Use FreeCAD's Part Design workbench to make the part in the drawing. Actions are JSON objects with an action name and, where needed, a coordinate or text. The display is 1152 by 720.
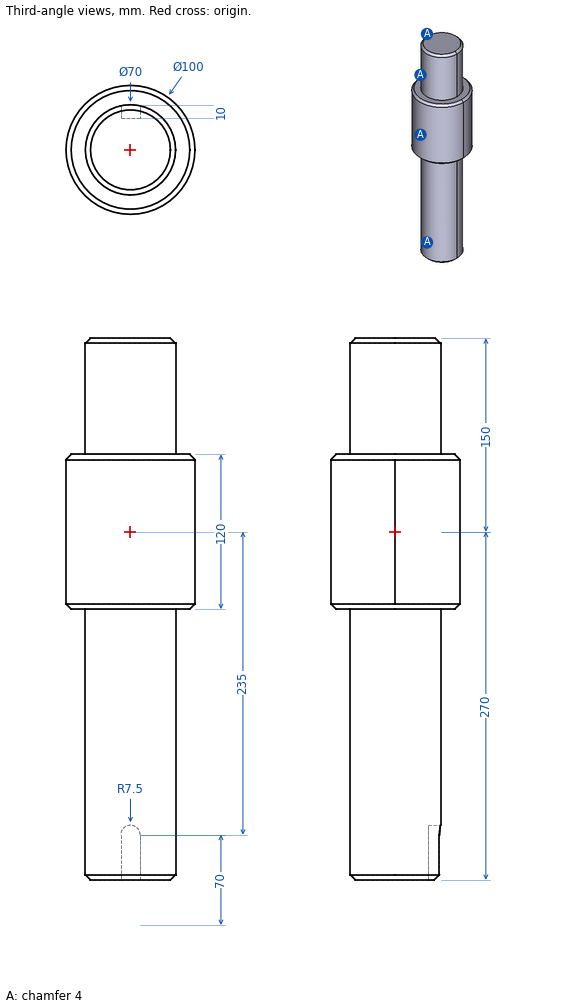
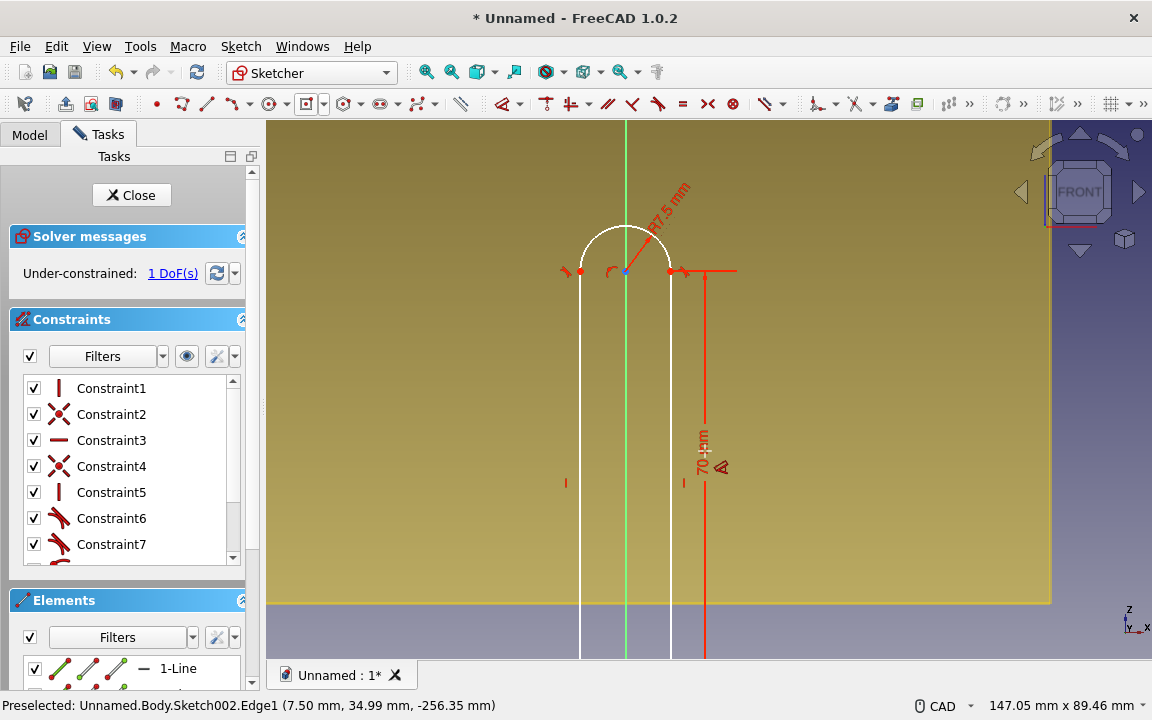
{"action": "left_click", "coordinate": [671, 271]}
{"action": "left_click", "coordinate": [705, 181]}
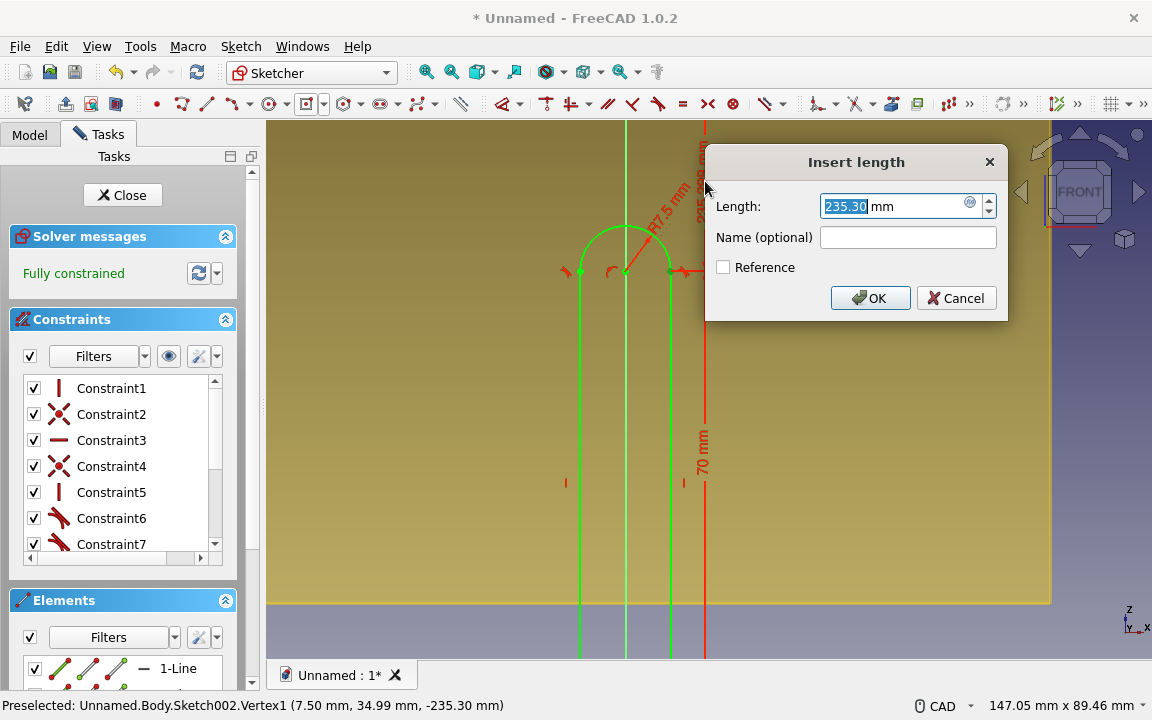
{"action": "type", "text": "235"}
{"action": "key", "text": "Return"}
{"action": "key", "text": "Escape"}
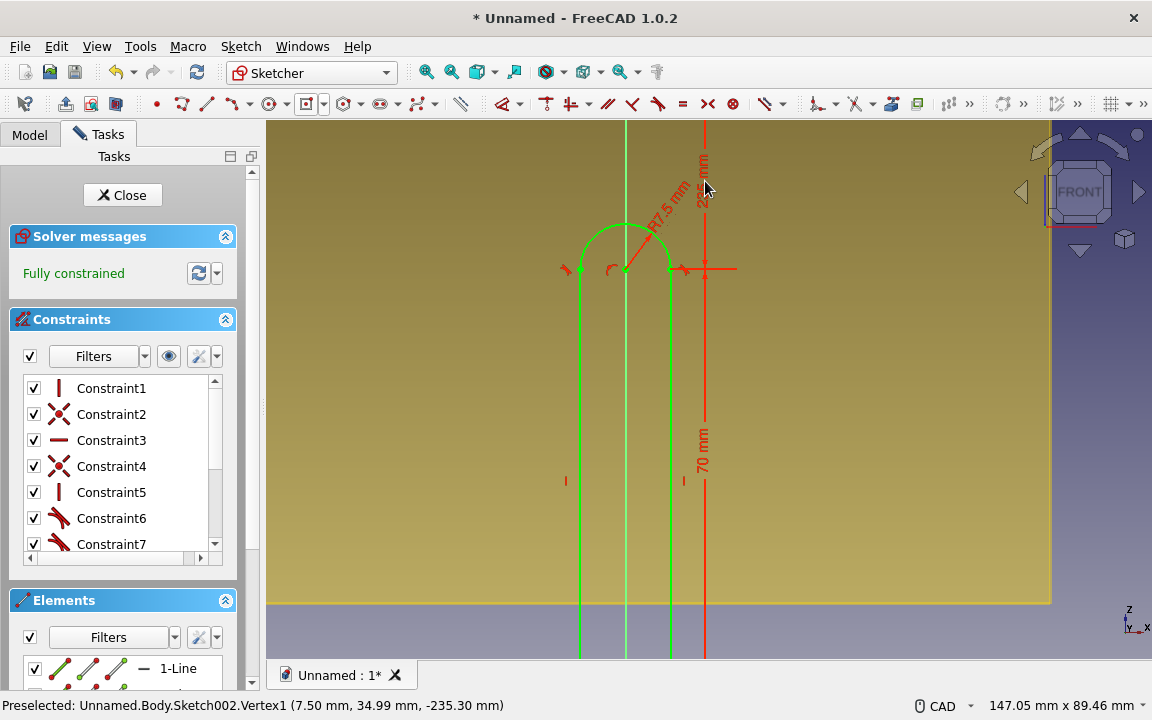
{"action": "left_click", "coordinate": [123, 195]}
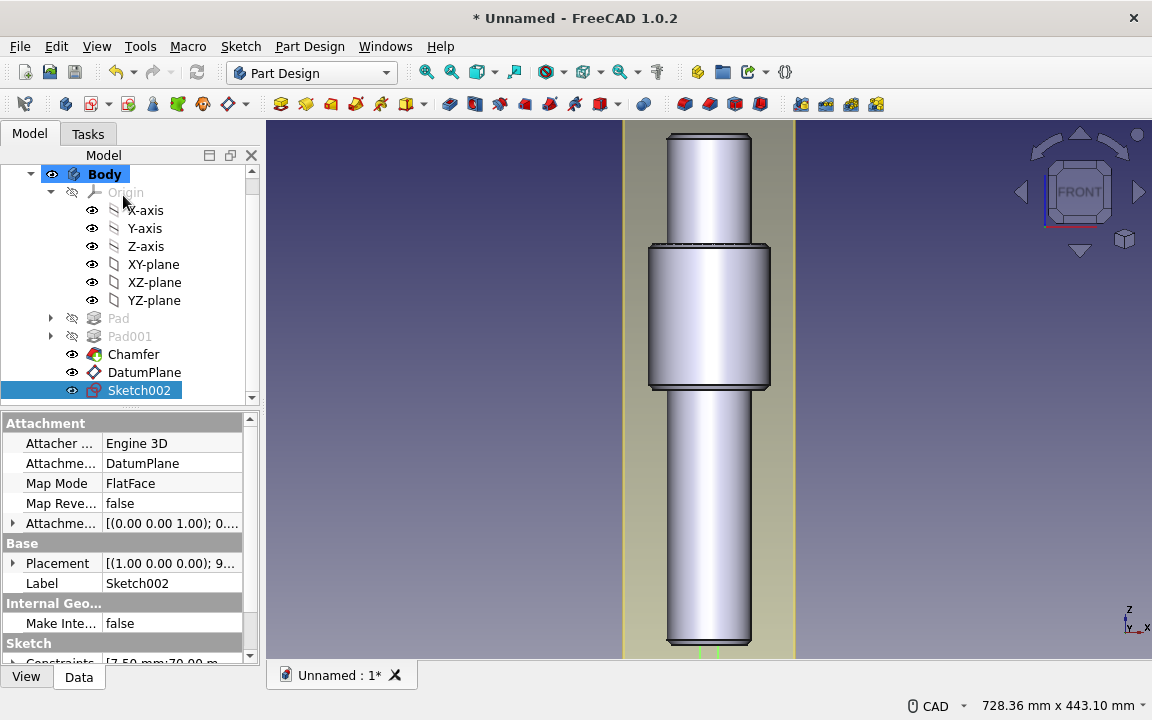
{"action": "left_click", "coordinate": [450, 104]}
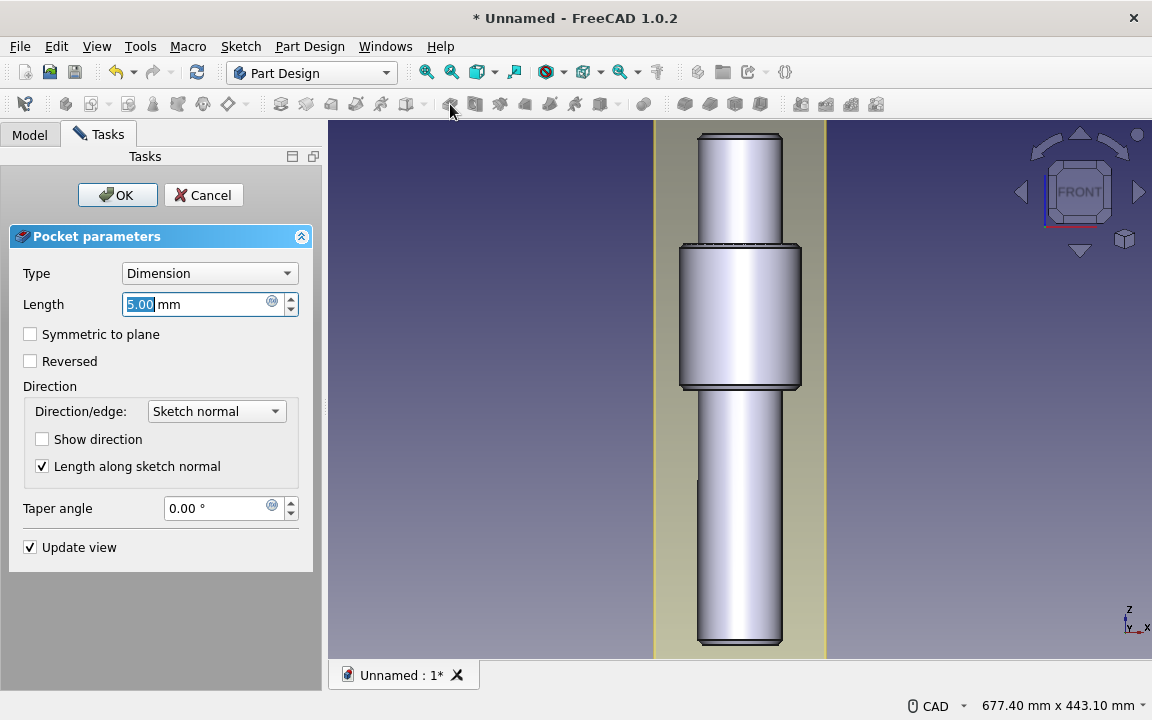
{"action": "type", "text": "10"}
{"action": "key", "text": "Tab"}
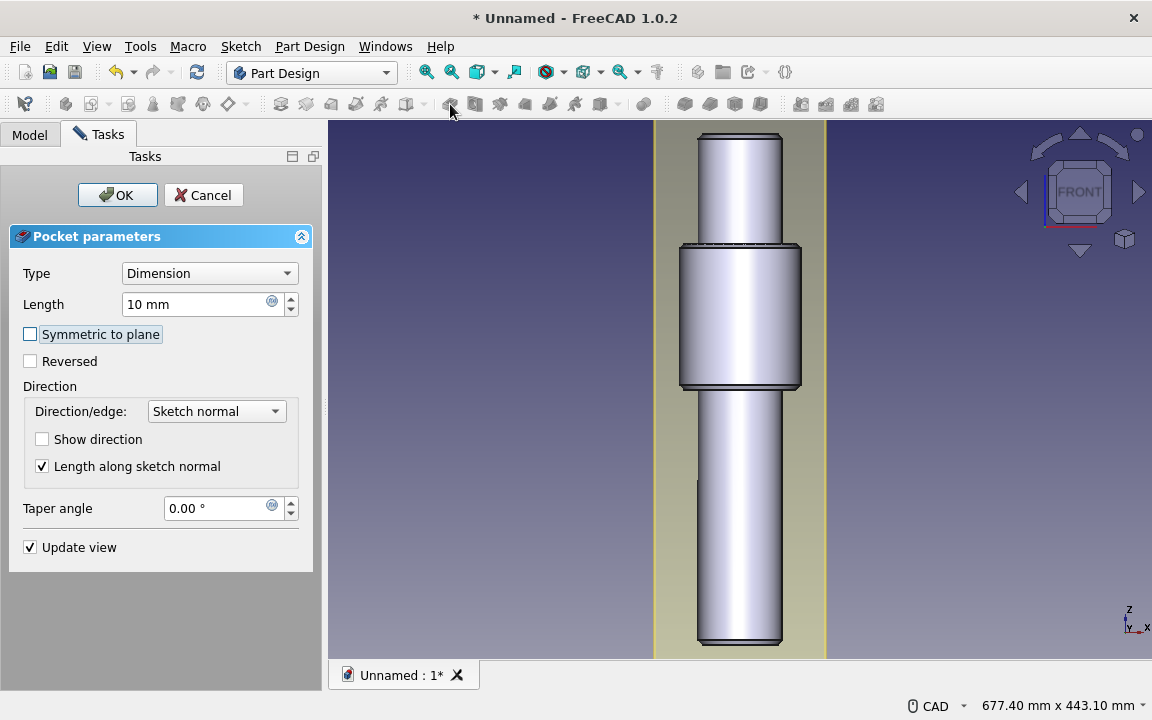
{"action": "left_click", "coordinate": [31, 361]}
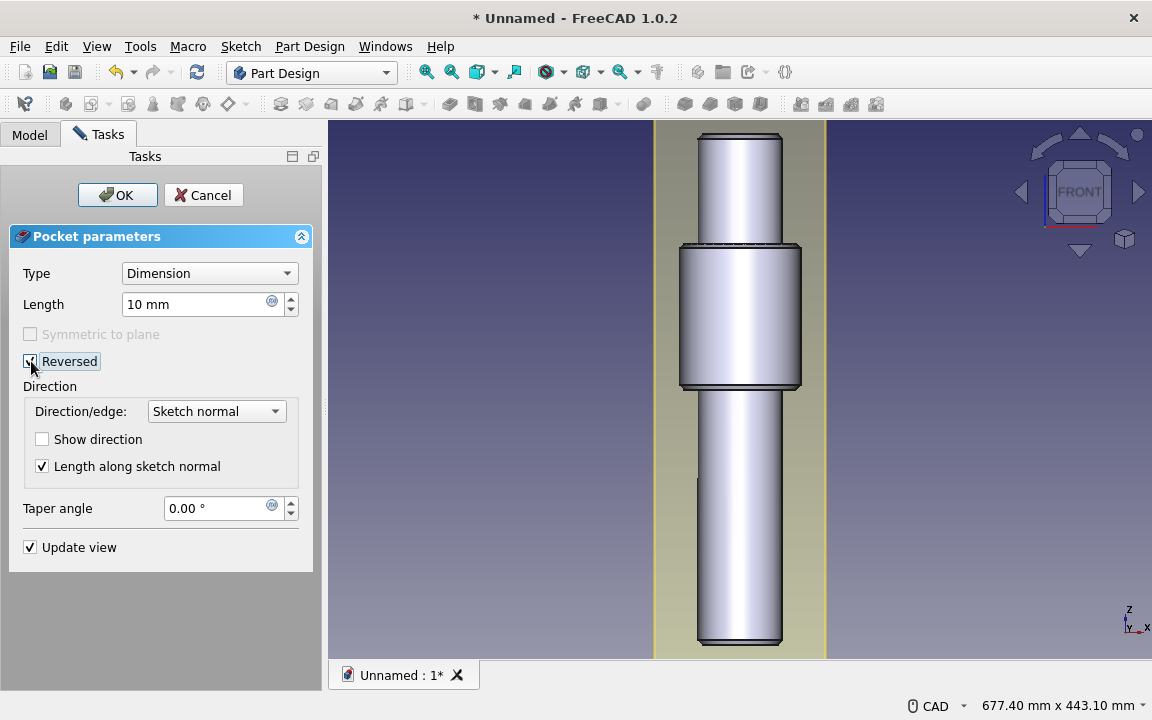
{"action": "left_click", "coordinate": [118, 195]}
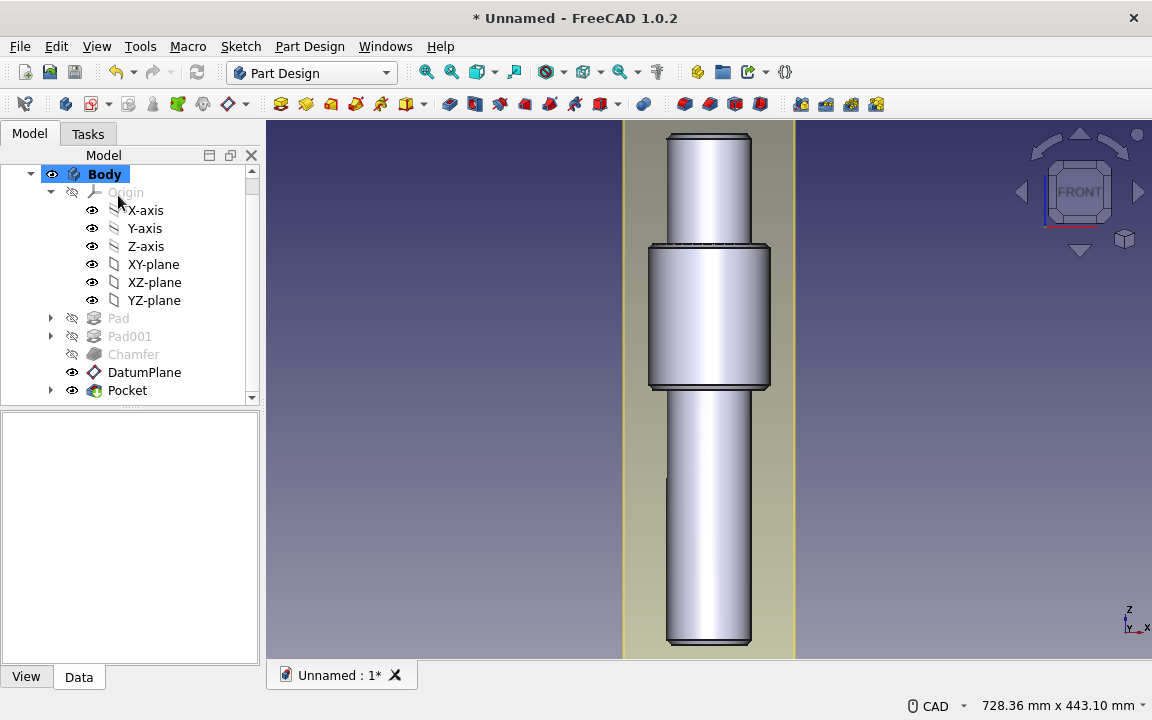
{"action": "left_click", "coordinate": [117, 372]}
{"action": "key", "text": "space"}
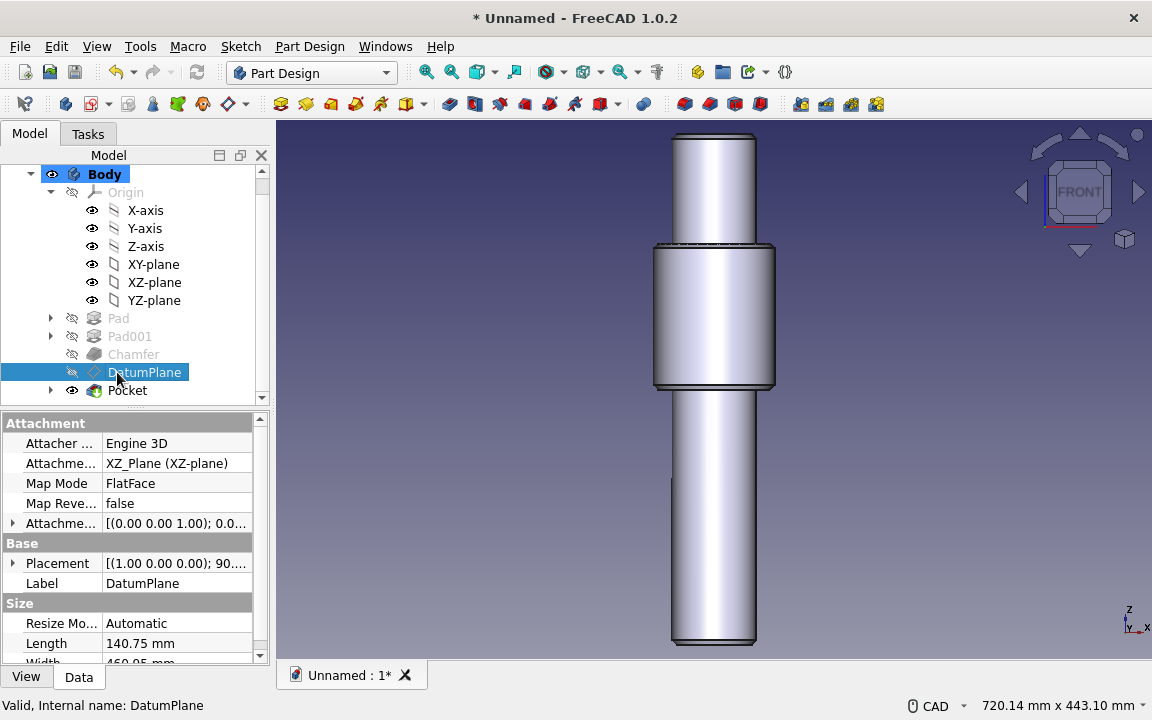
{"action": "key", "text": "0"}